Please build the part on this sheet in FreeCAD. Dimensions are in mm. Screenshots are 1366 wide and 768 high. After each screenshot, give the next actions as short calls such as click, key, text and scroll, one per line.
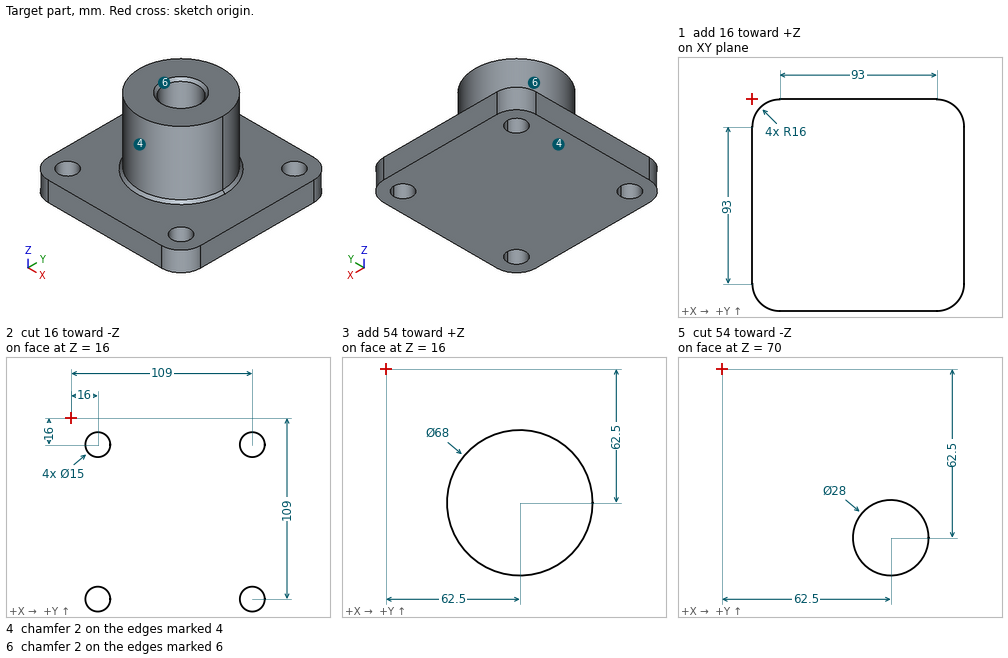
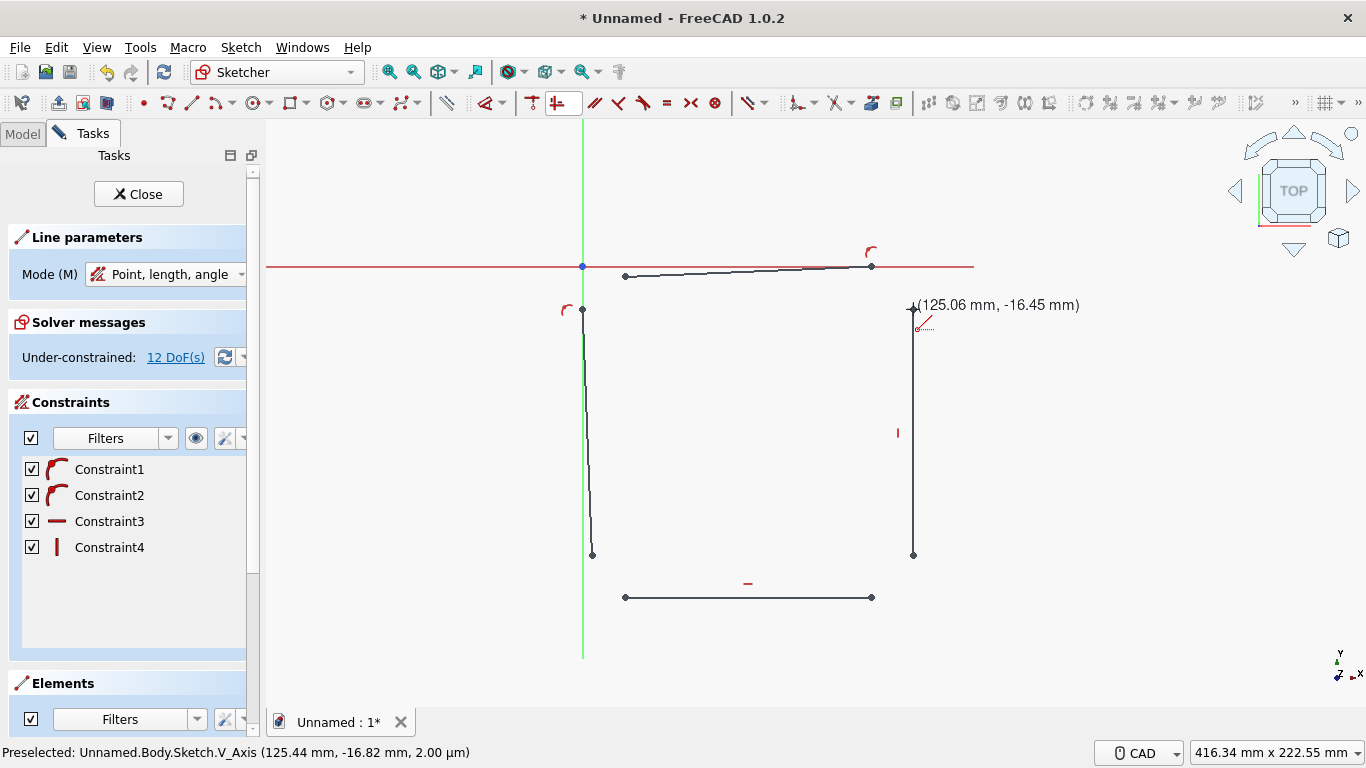
key(g)
key(3)
key(a)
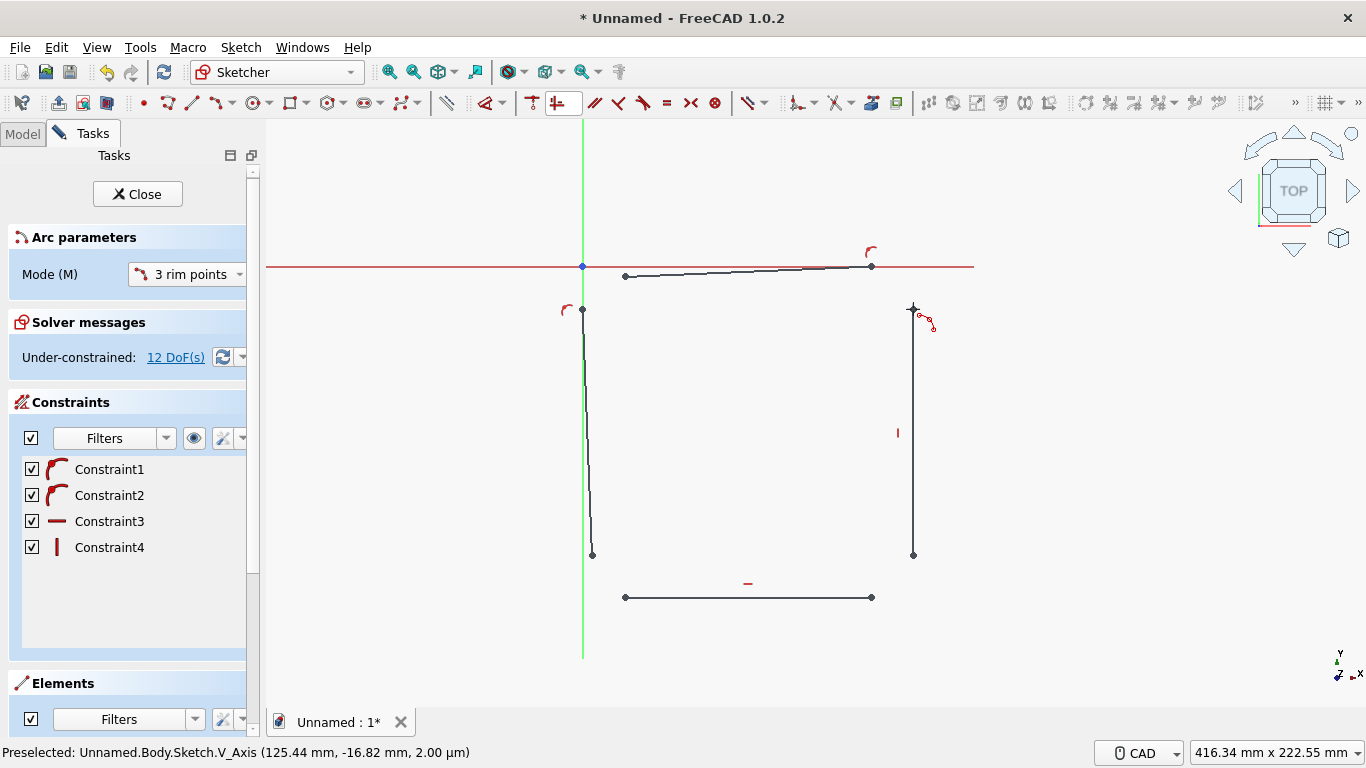
click(625, 277)
click(583, 310)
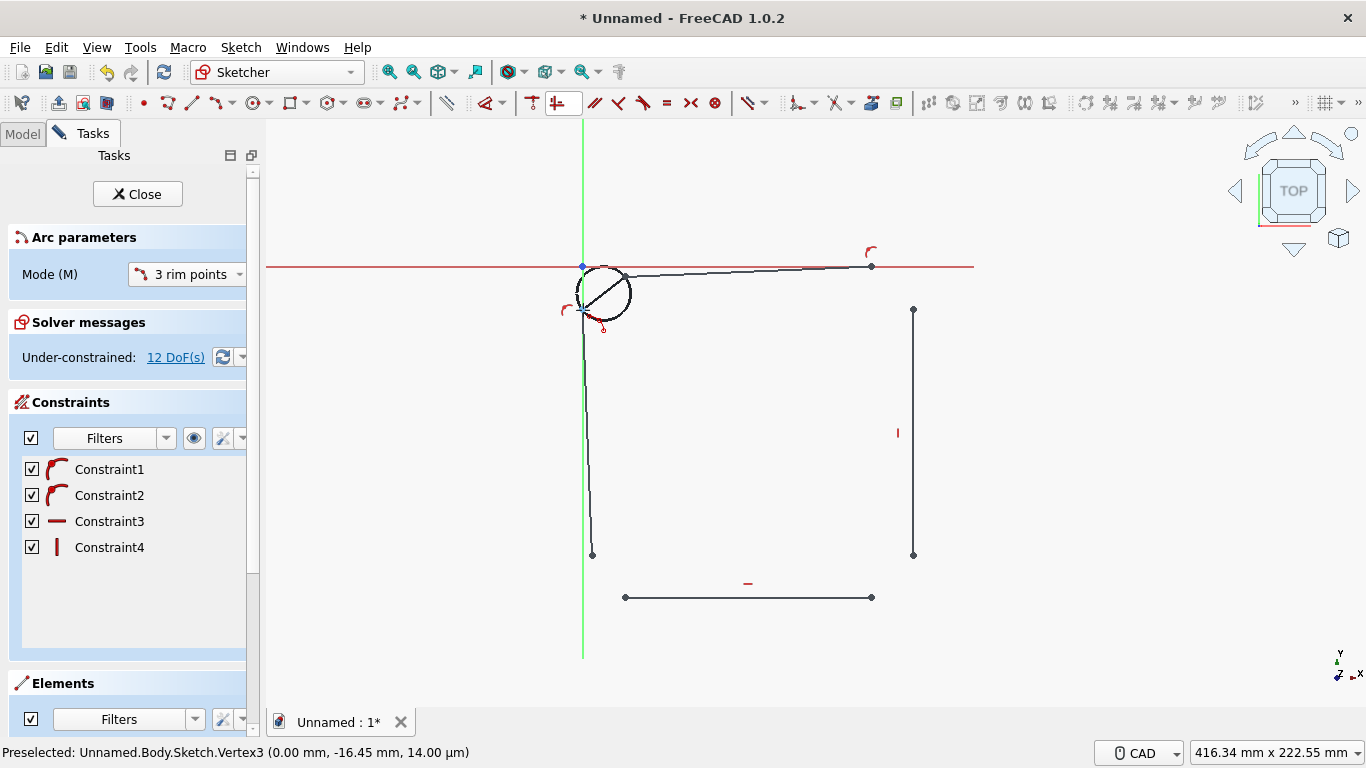
scroll(595, 279, up, 2)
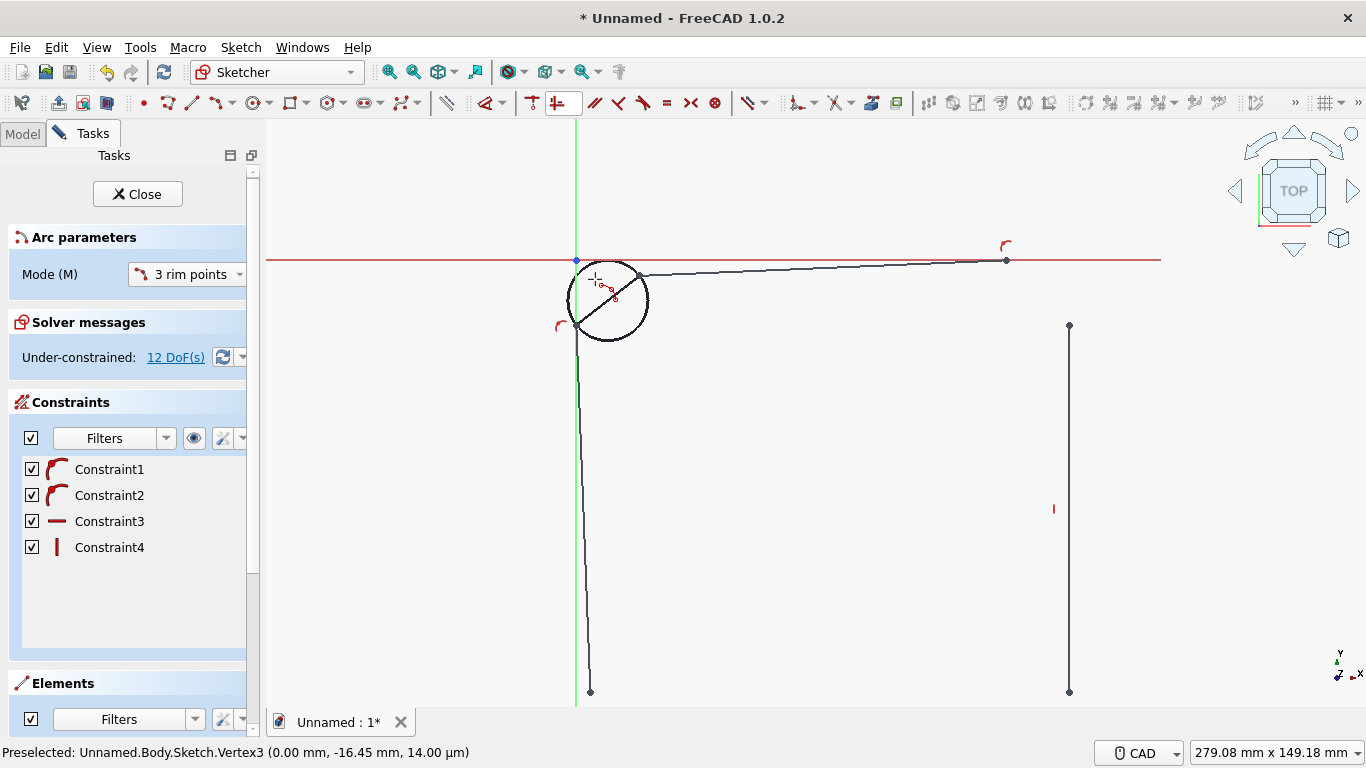
click(595, 279)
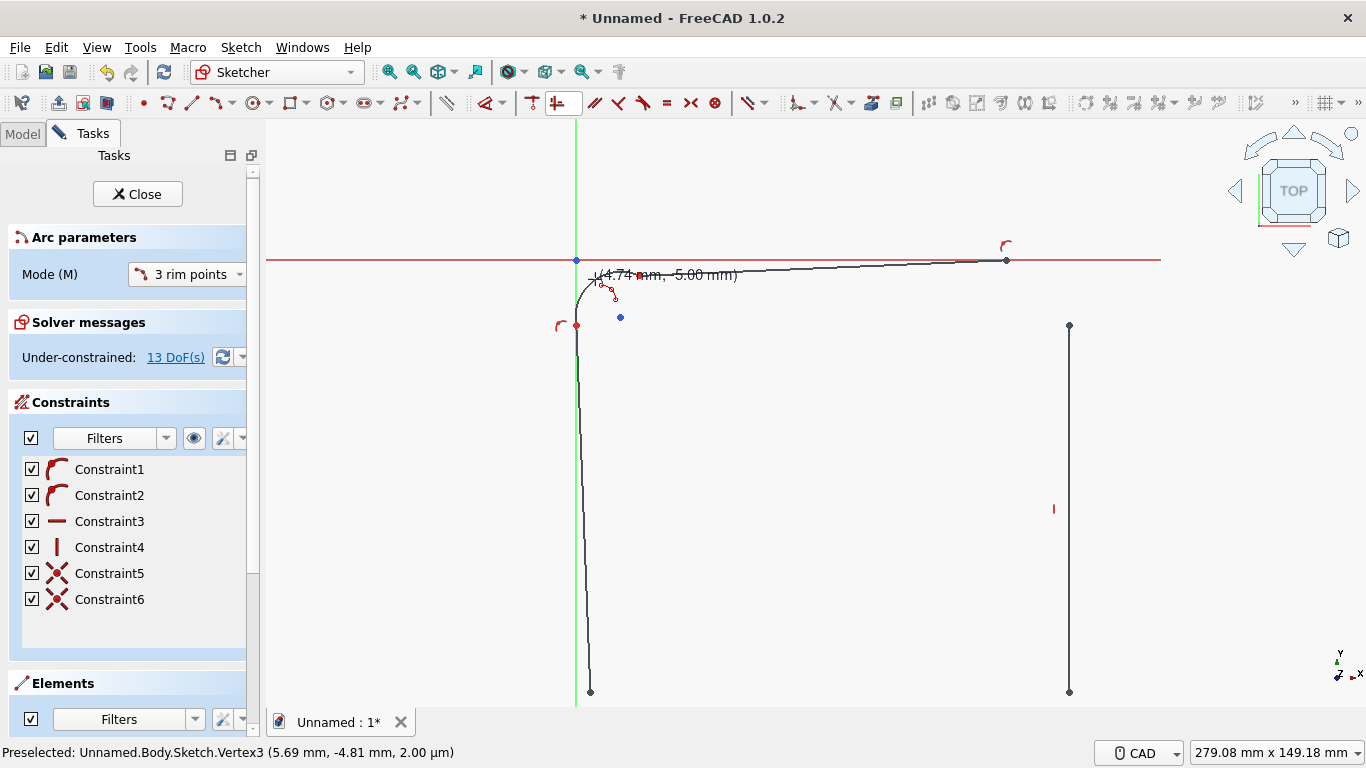
scroll(408, 147, down, 1)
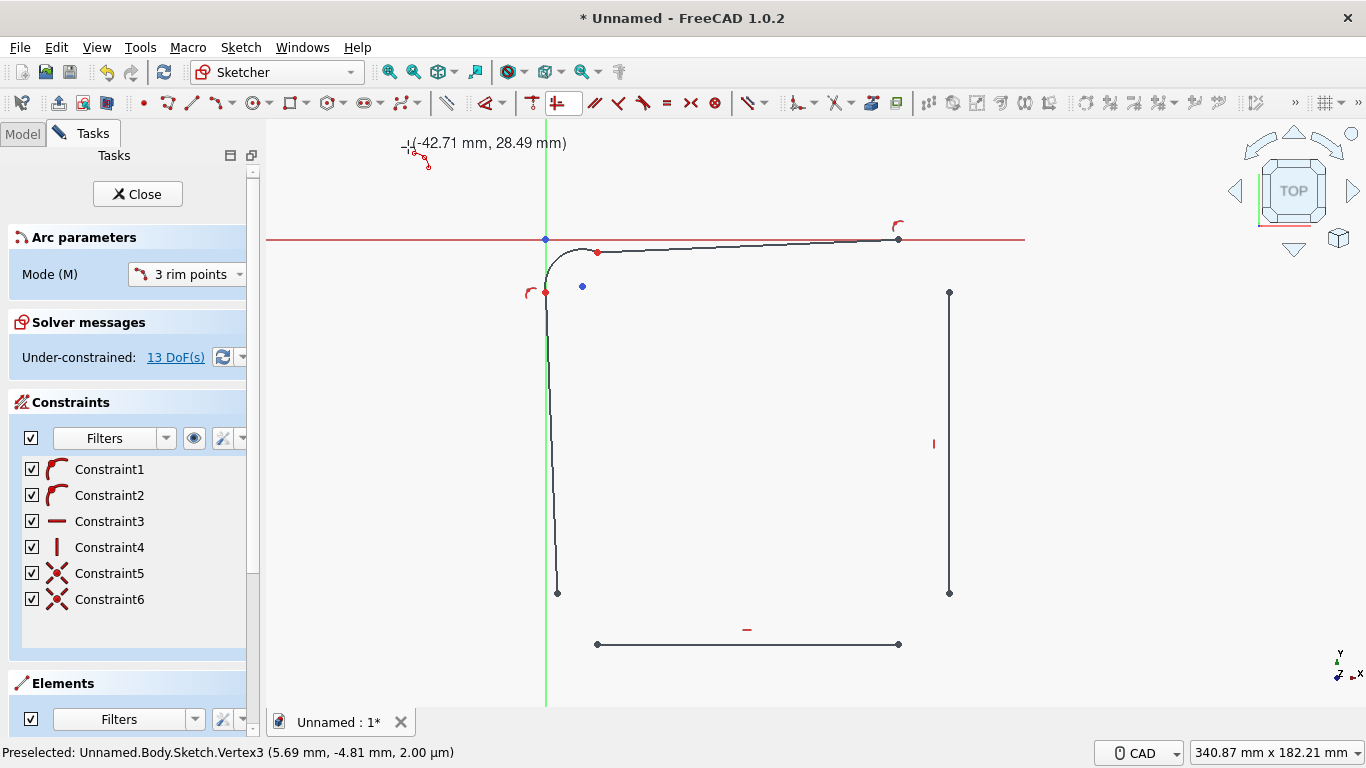
click(557, 593)
click(598, 645)
click(561, 628)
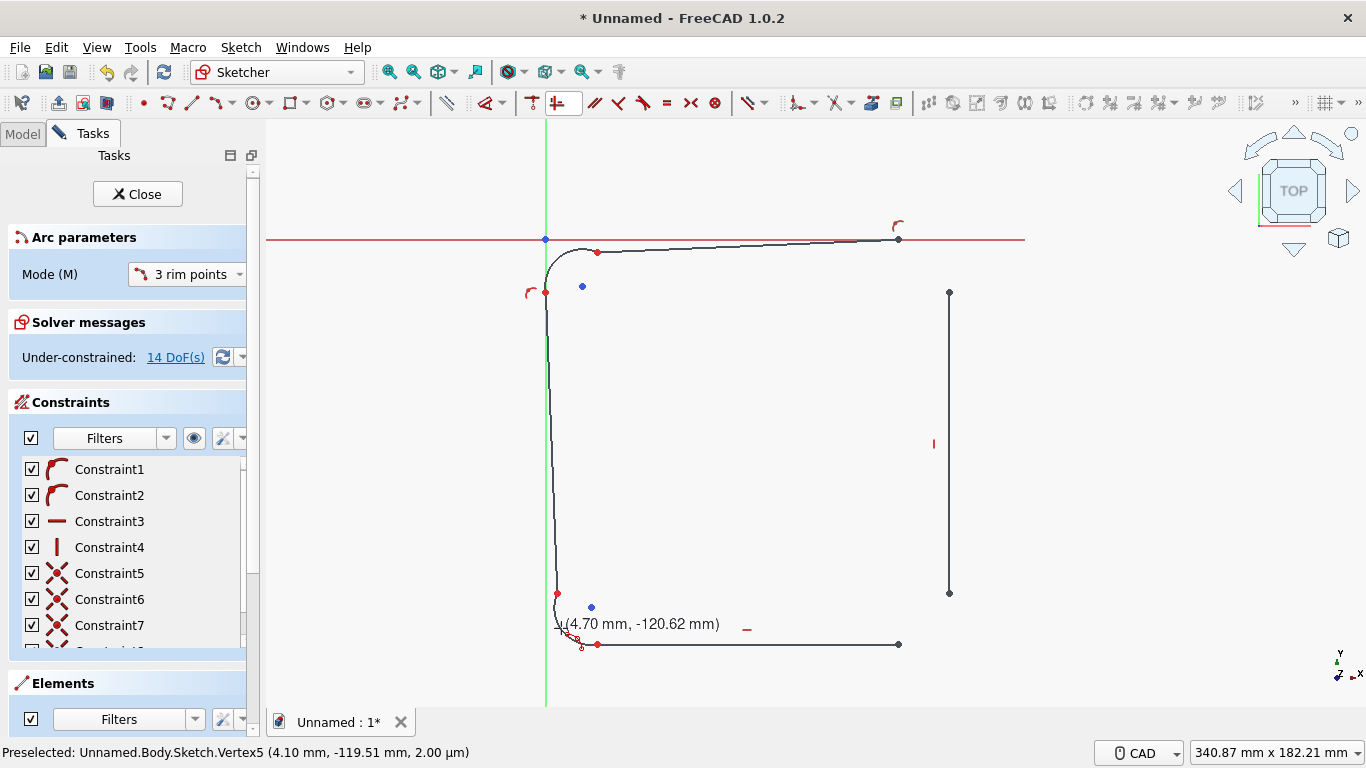
click(898, 645)
click(949, 593)
click(934, 628)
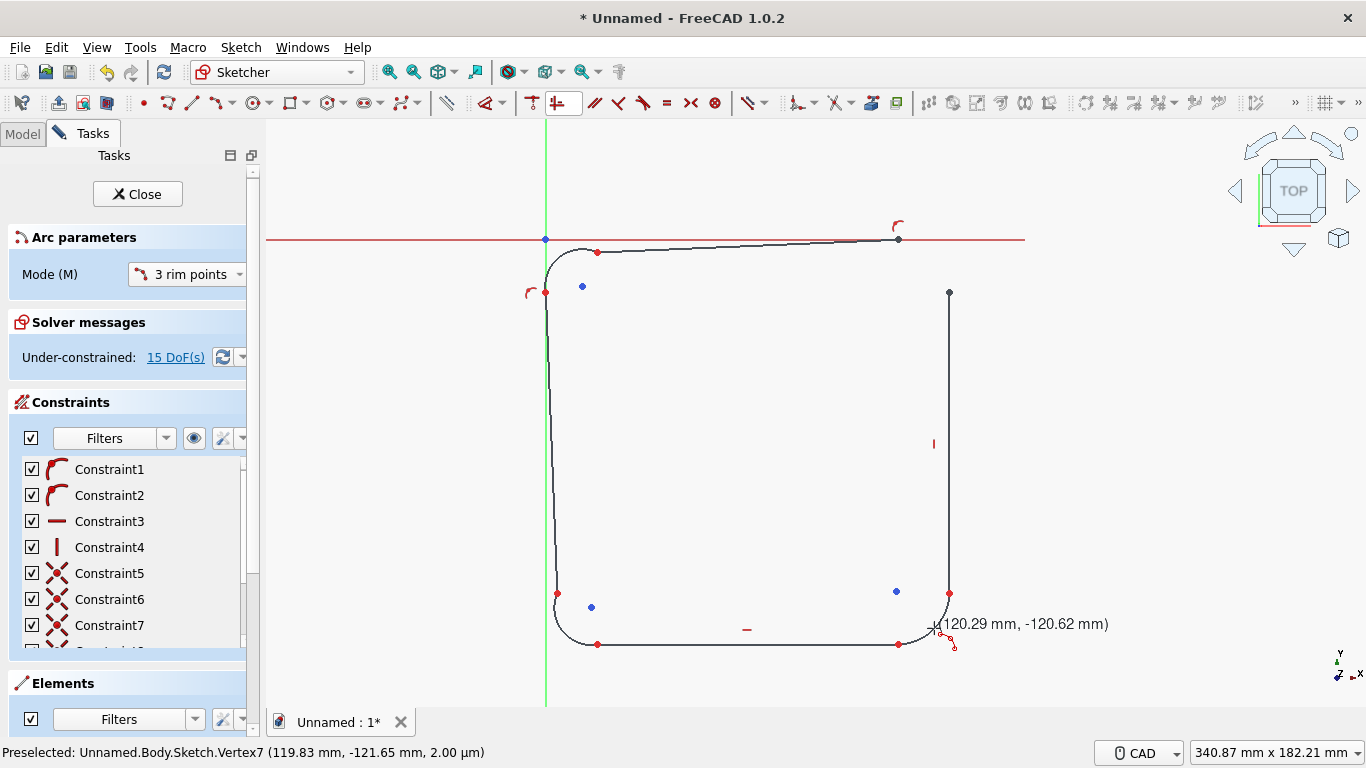
click(949, 293)
click(898, 240)
click(934, 255)
key(Escape)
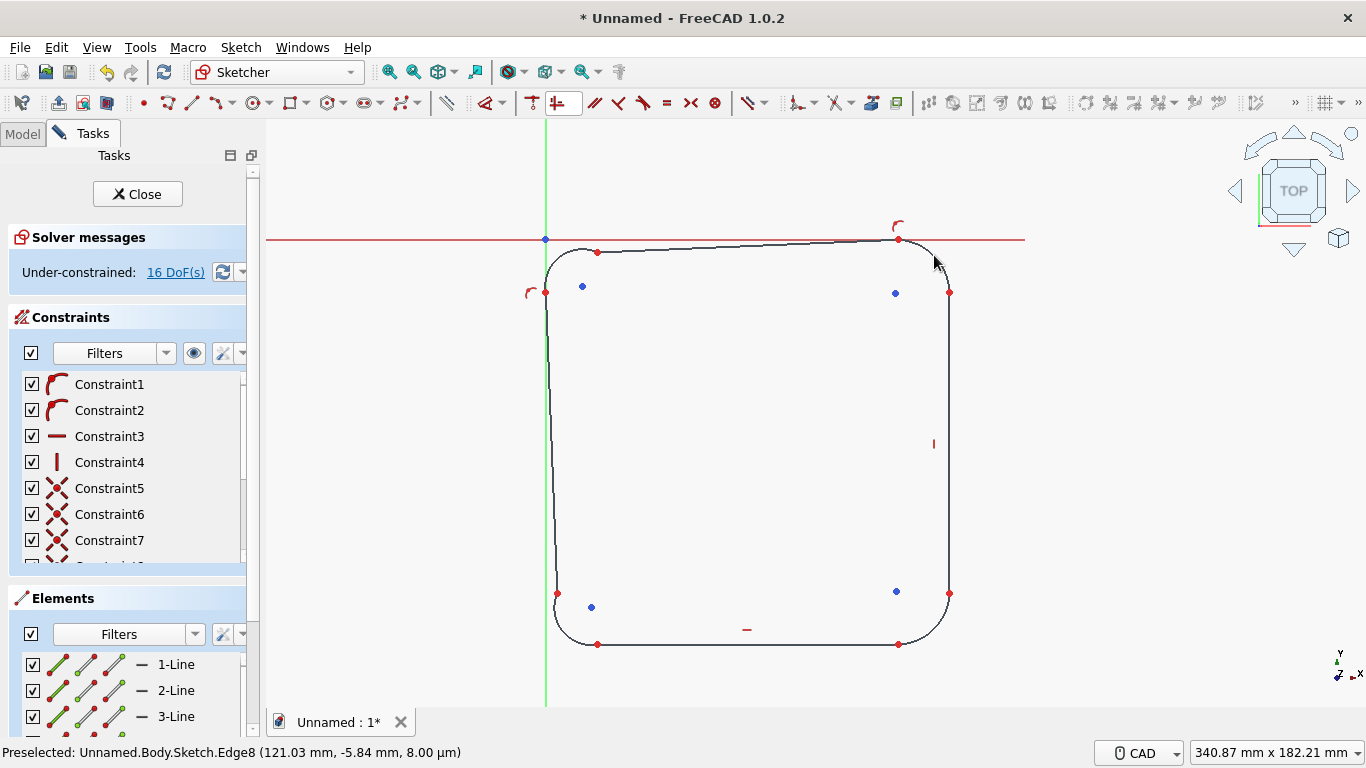
click(808, 244)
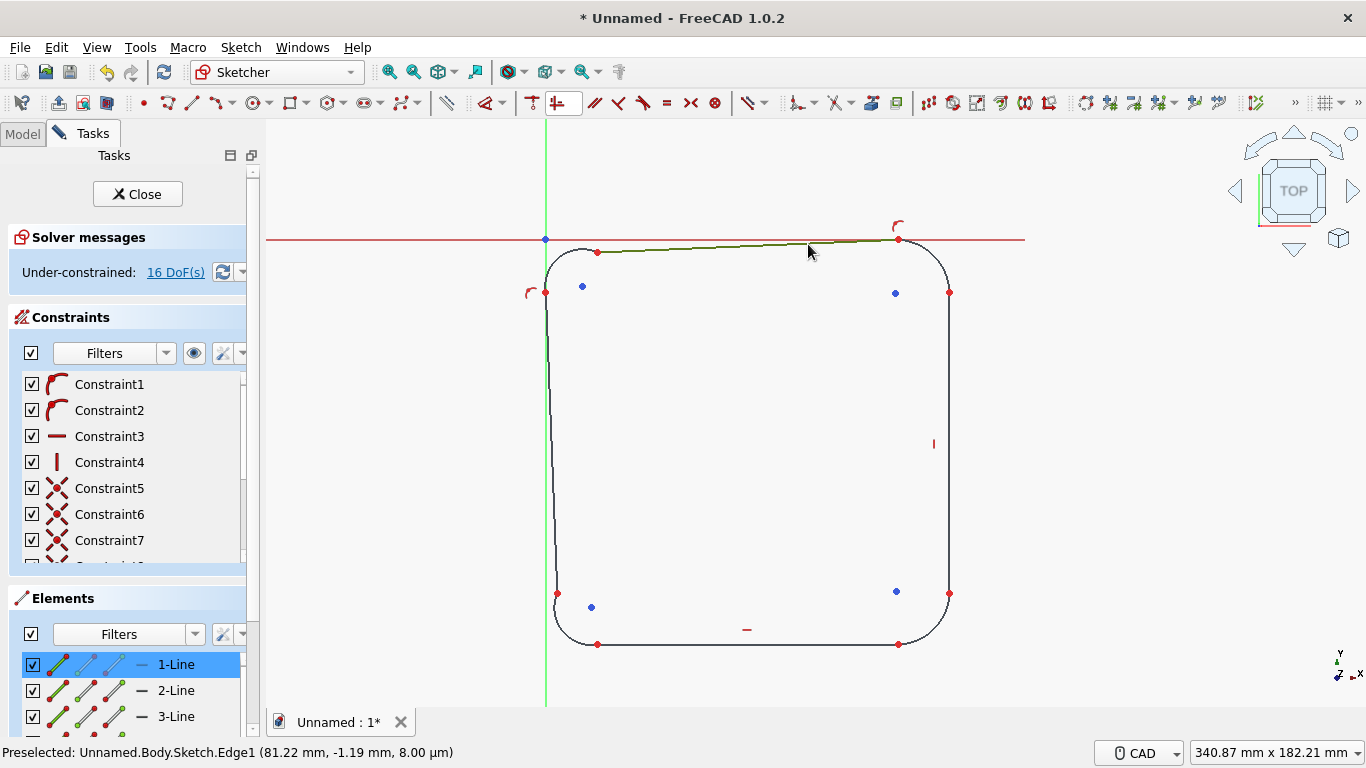
scroll(574, 250, up, 2)